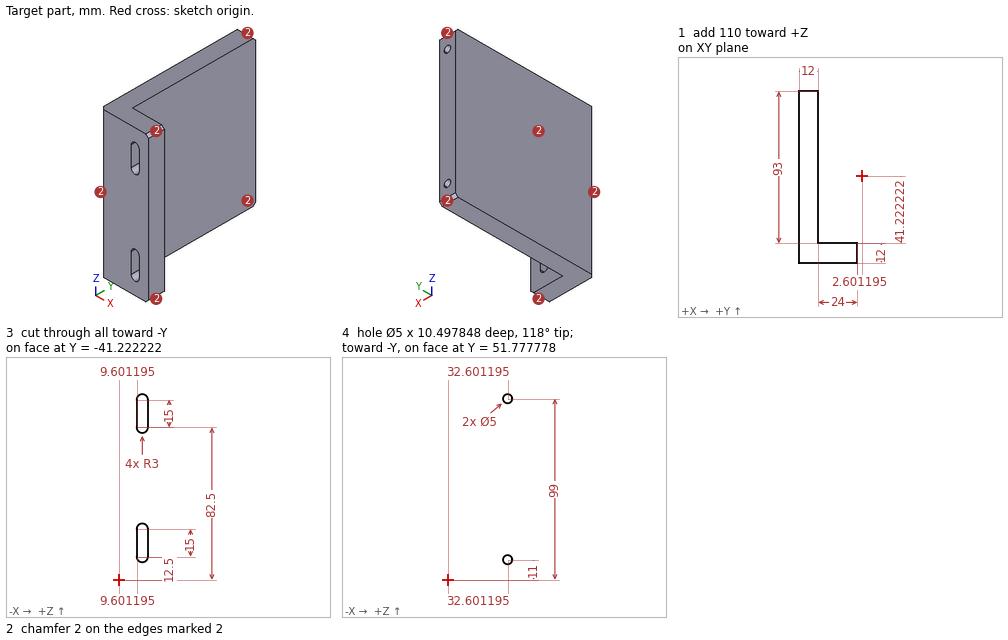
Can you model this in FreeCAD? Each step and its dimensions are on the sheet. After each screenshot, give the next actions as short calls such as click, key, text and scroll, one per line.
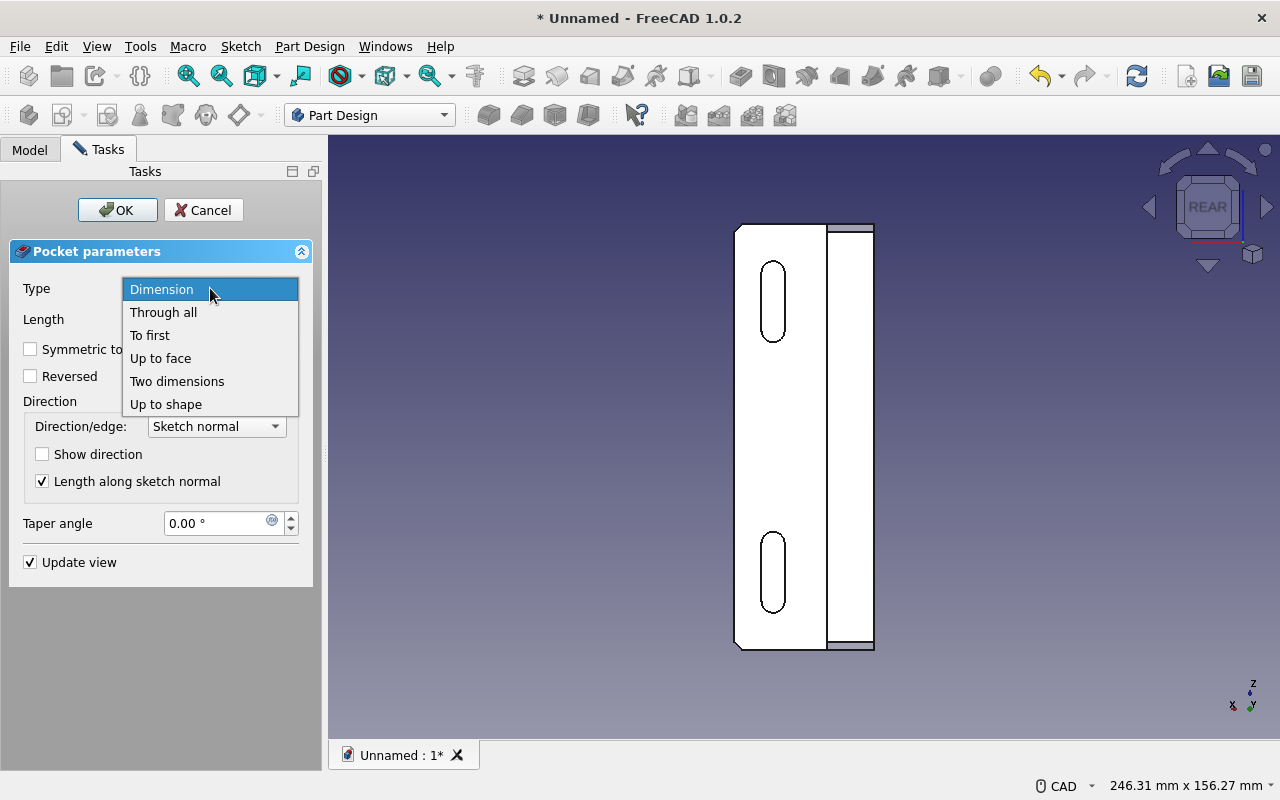
click(208, 312)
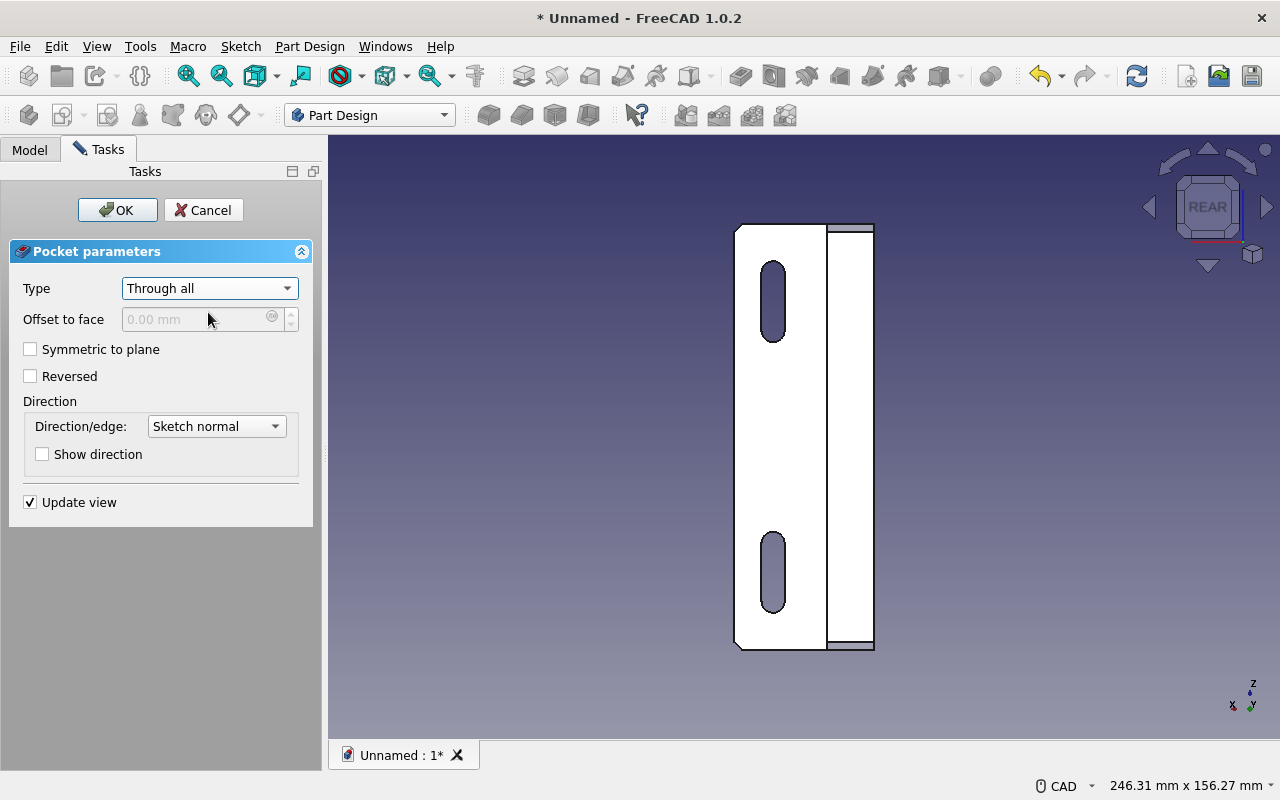
click(118, 210)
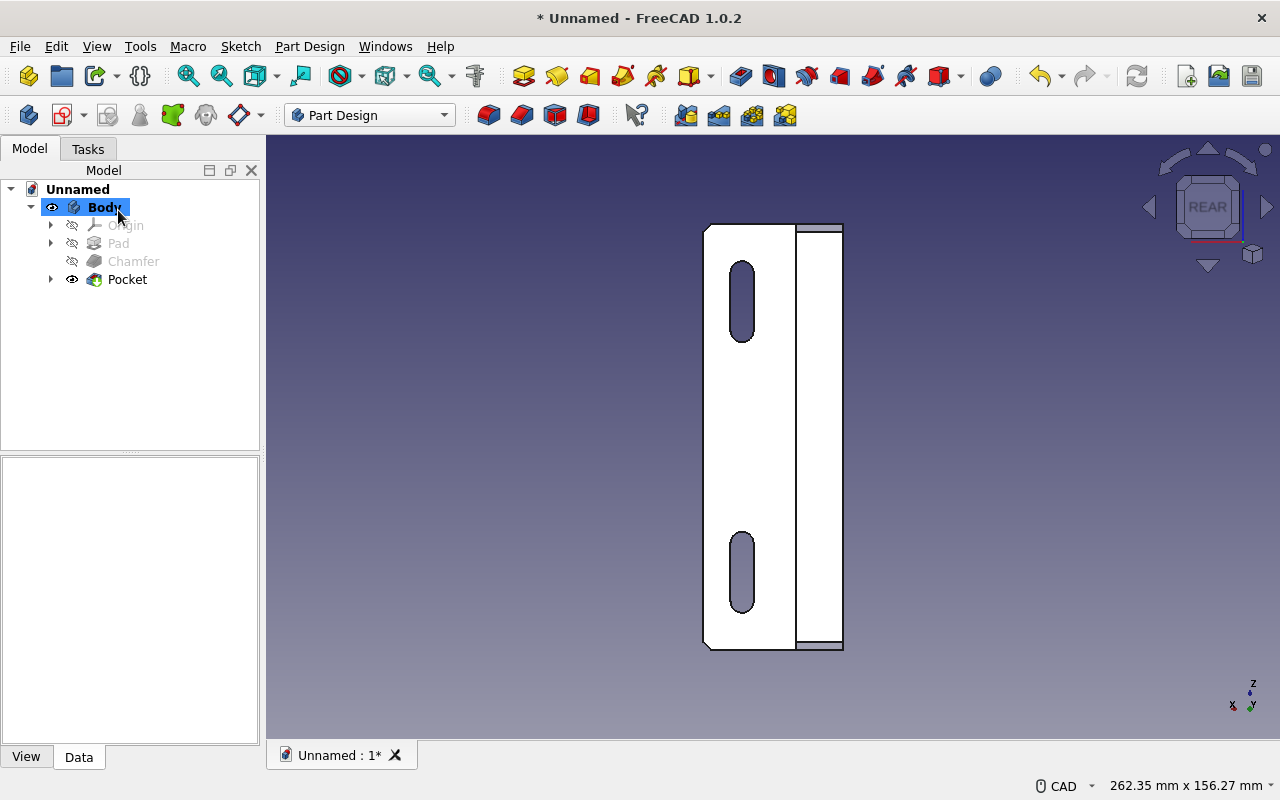
click(819, 260)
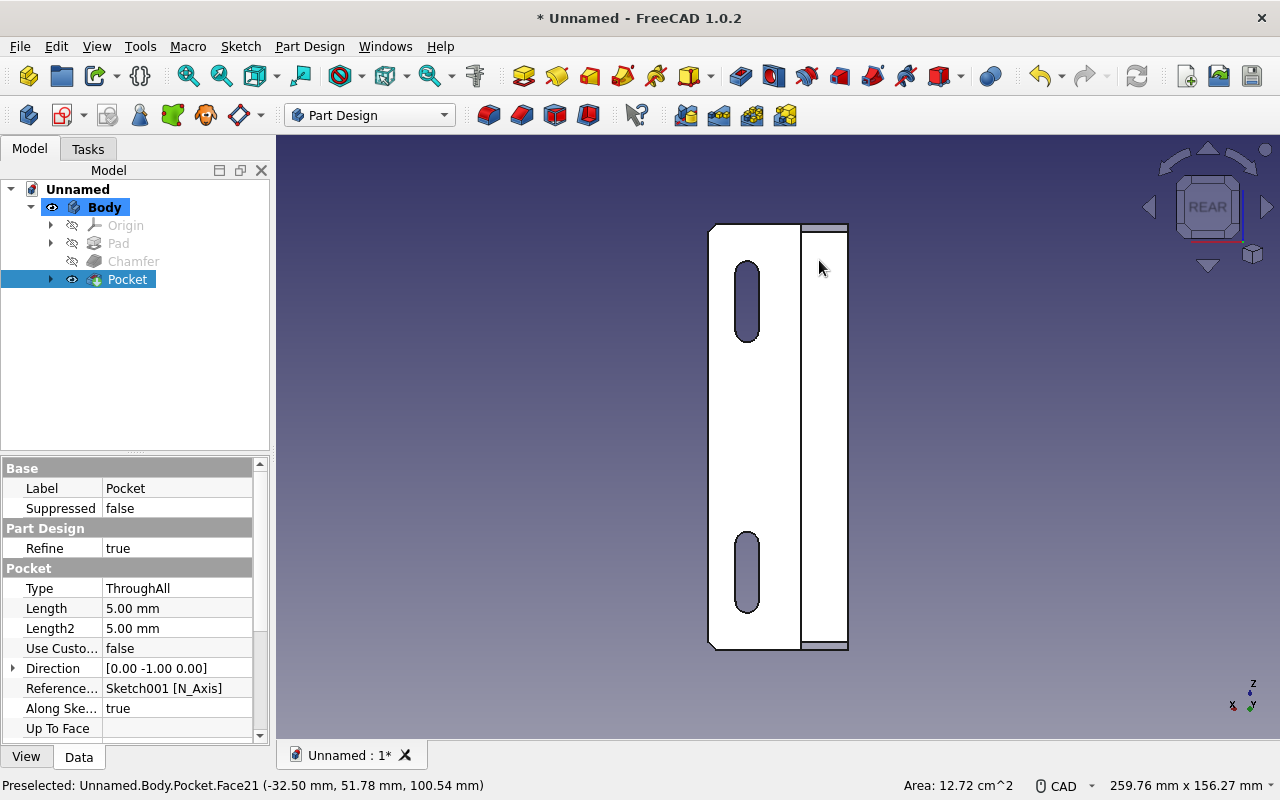
click(62, 116)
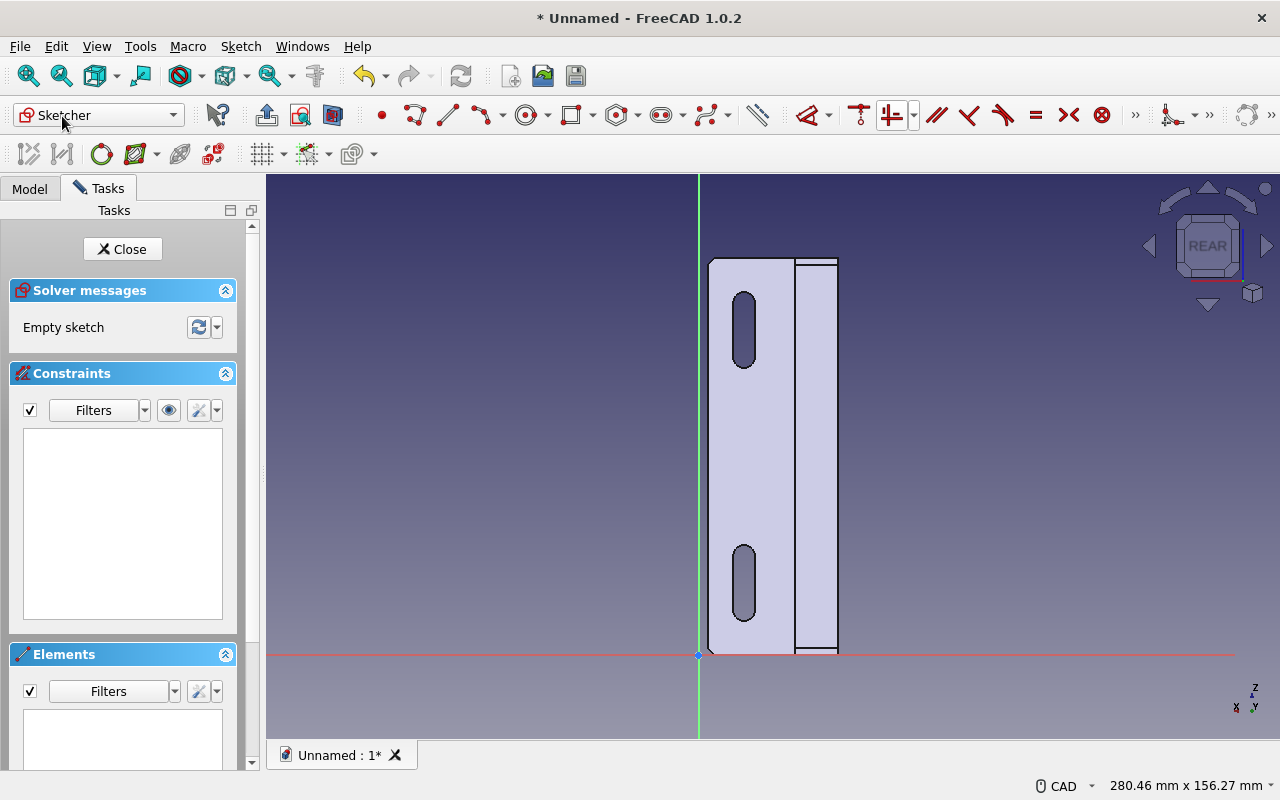
click(526, 116)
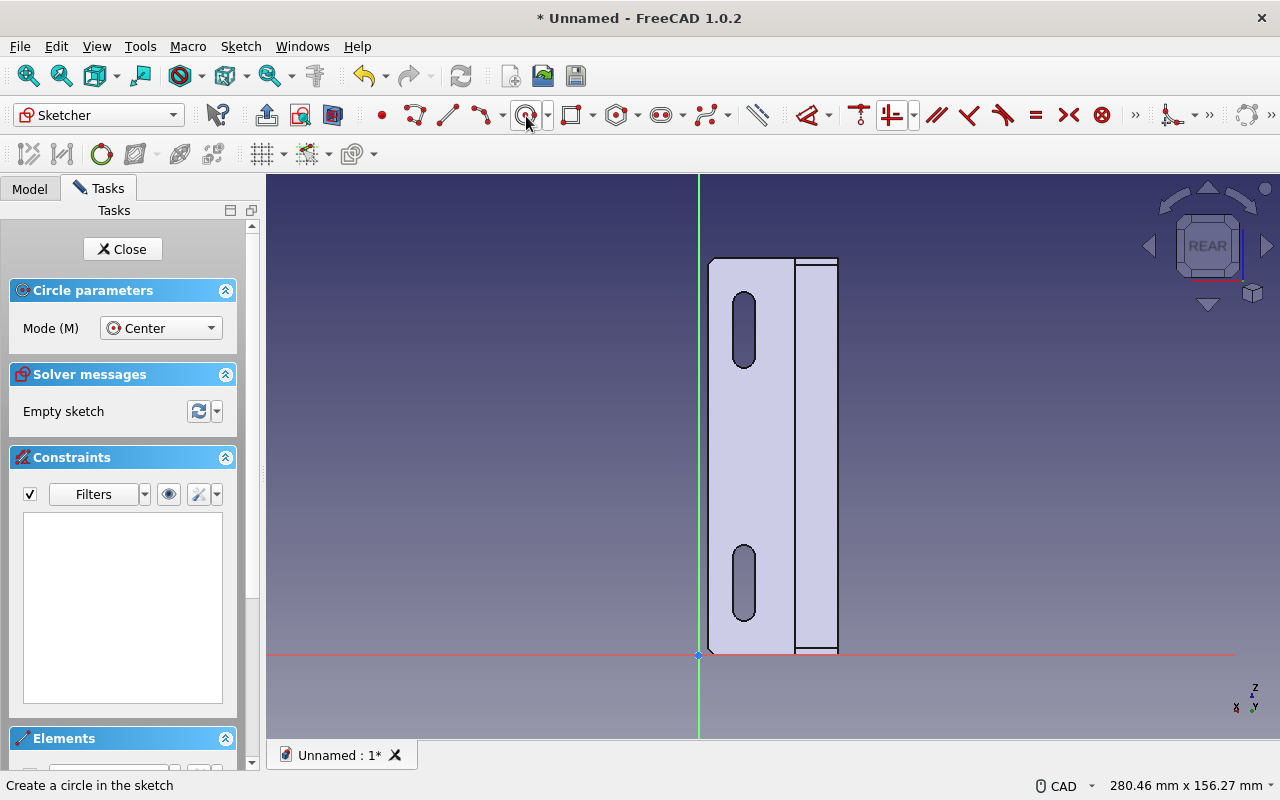
scroll(816, 297, up, 5)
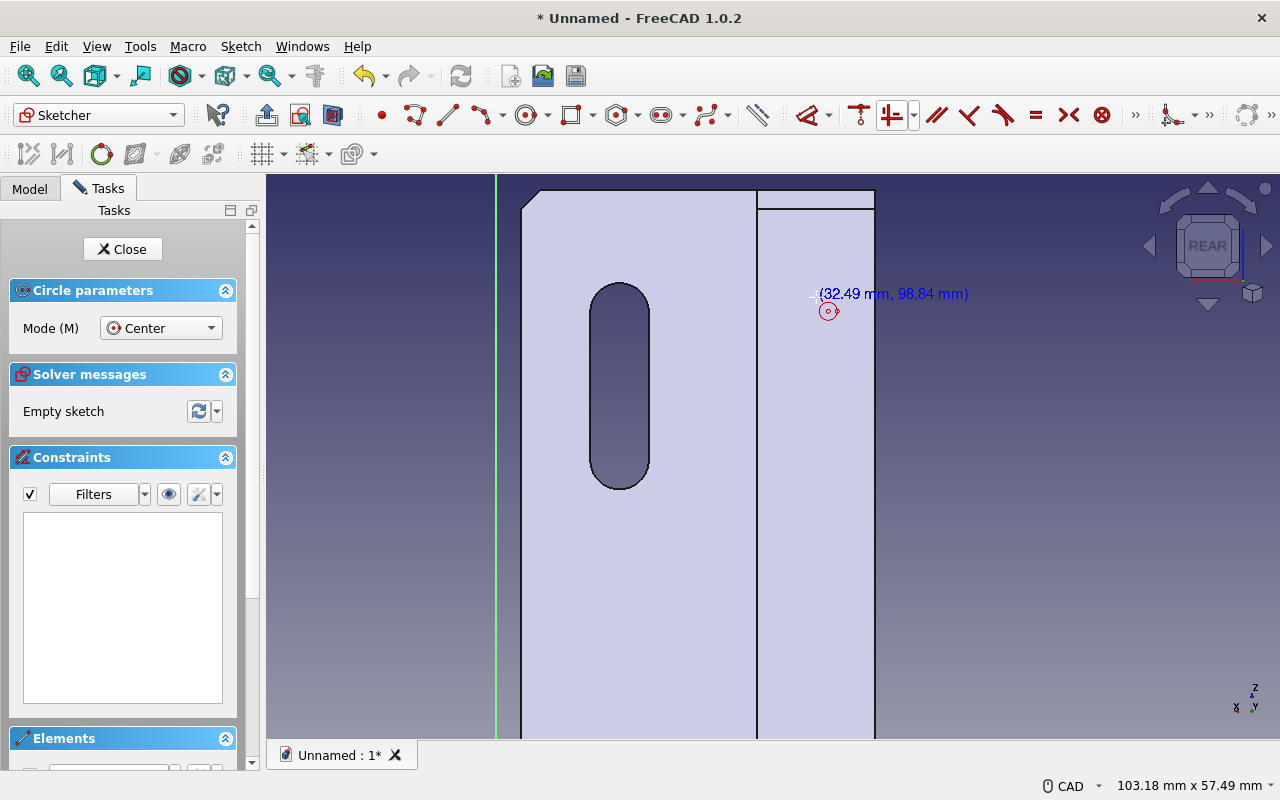
click(816, 298)
move(833, 280)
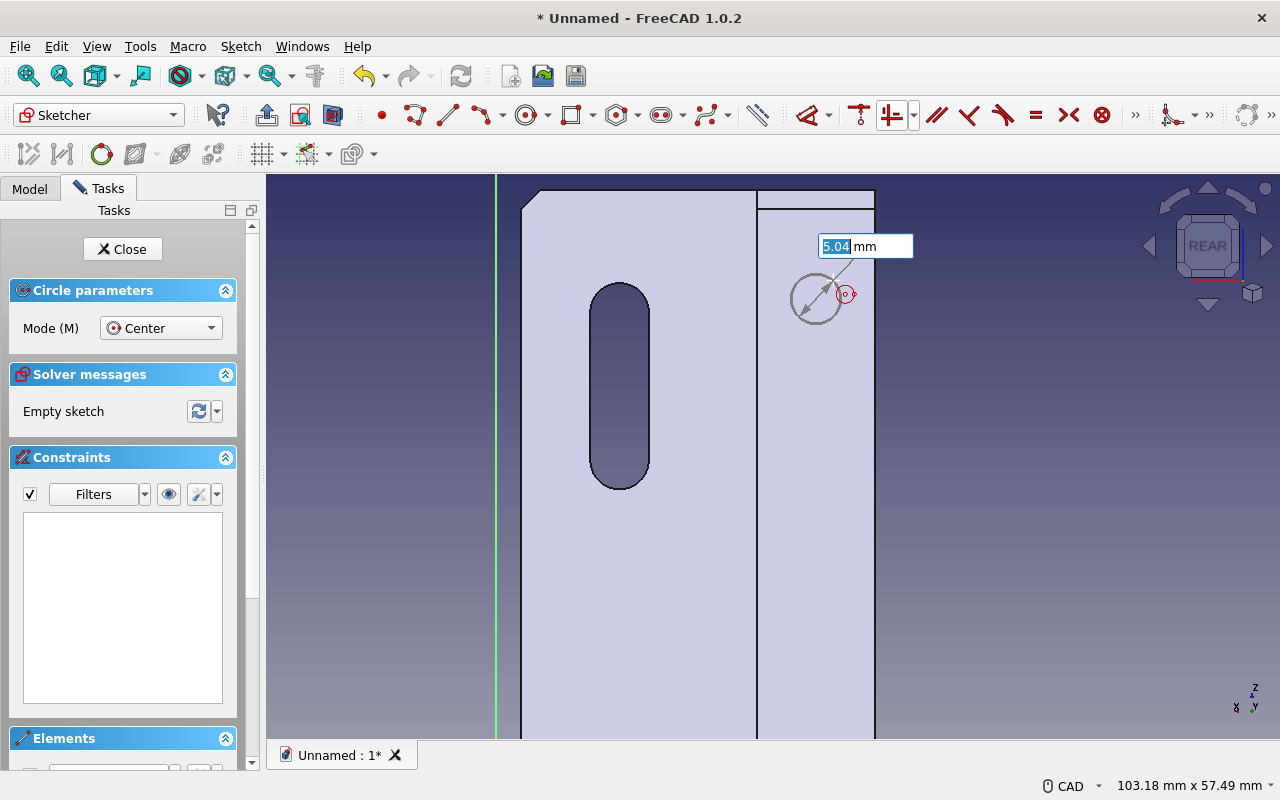
text(5)
key(Return)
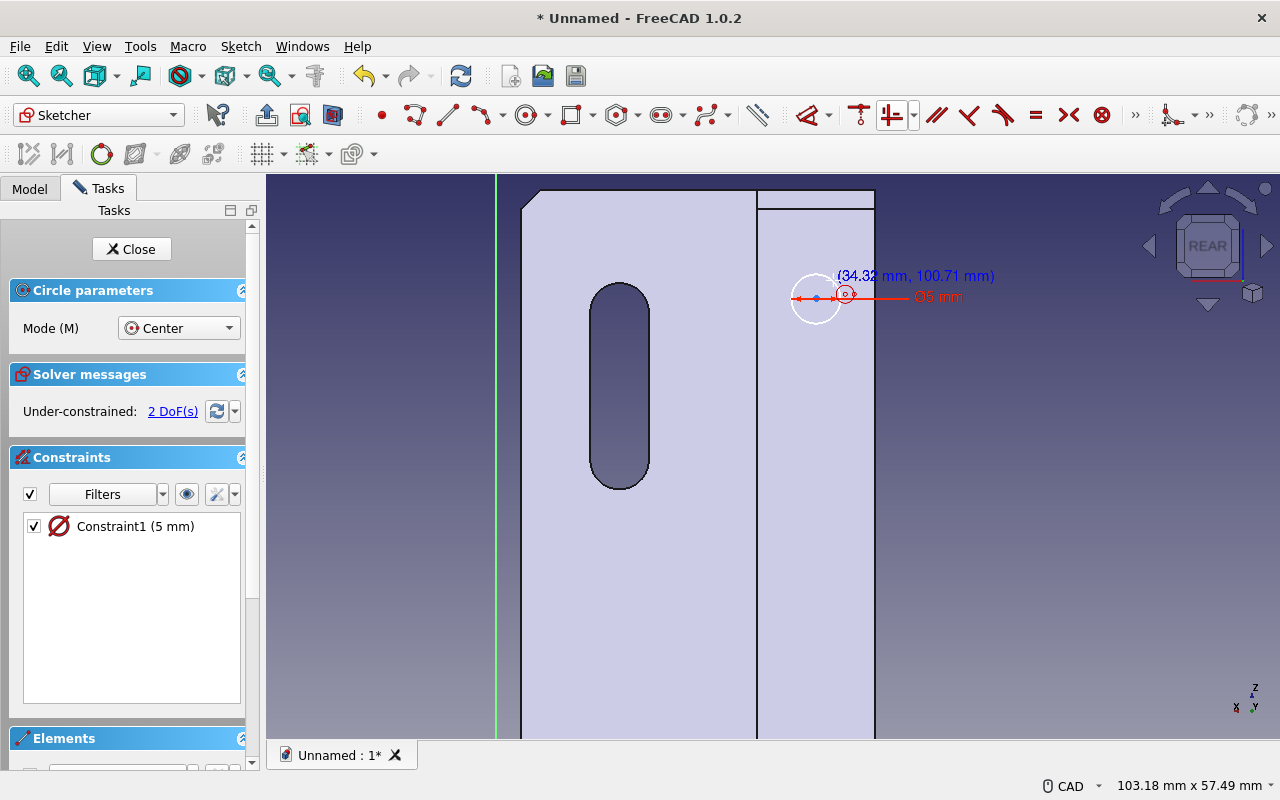
scroll(726, 273, down, 5)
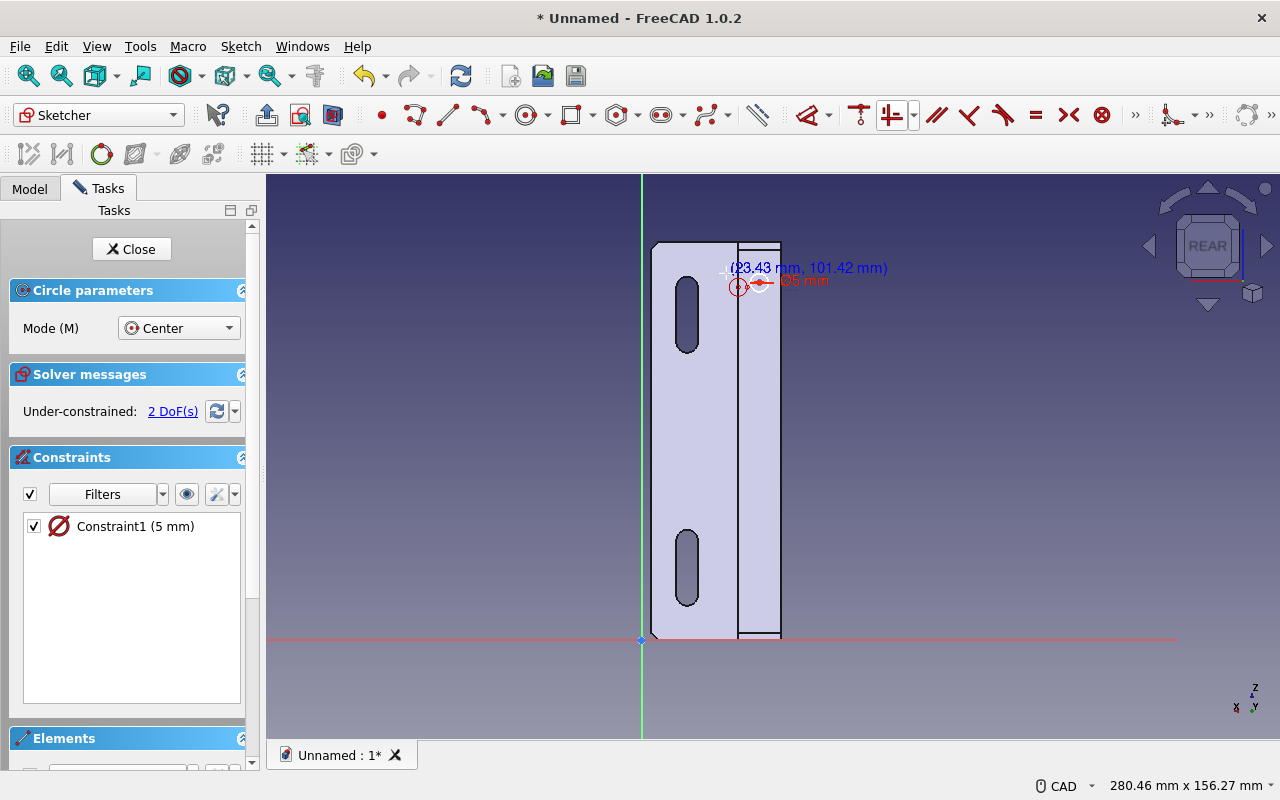
scroll(759, 600, up, 5)